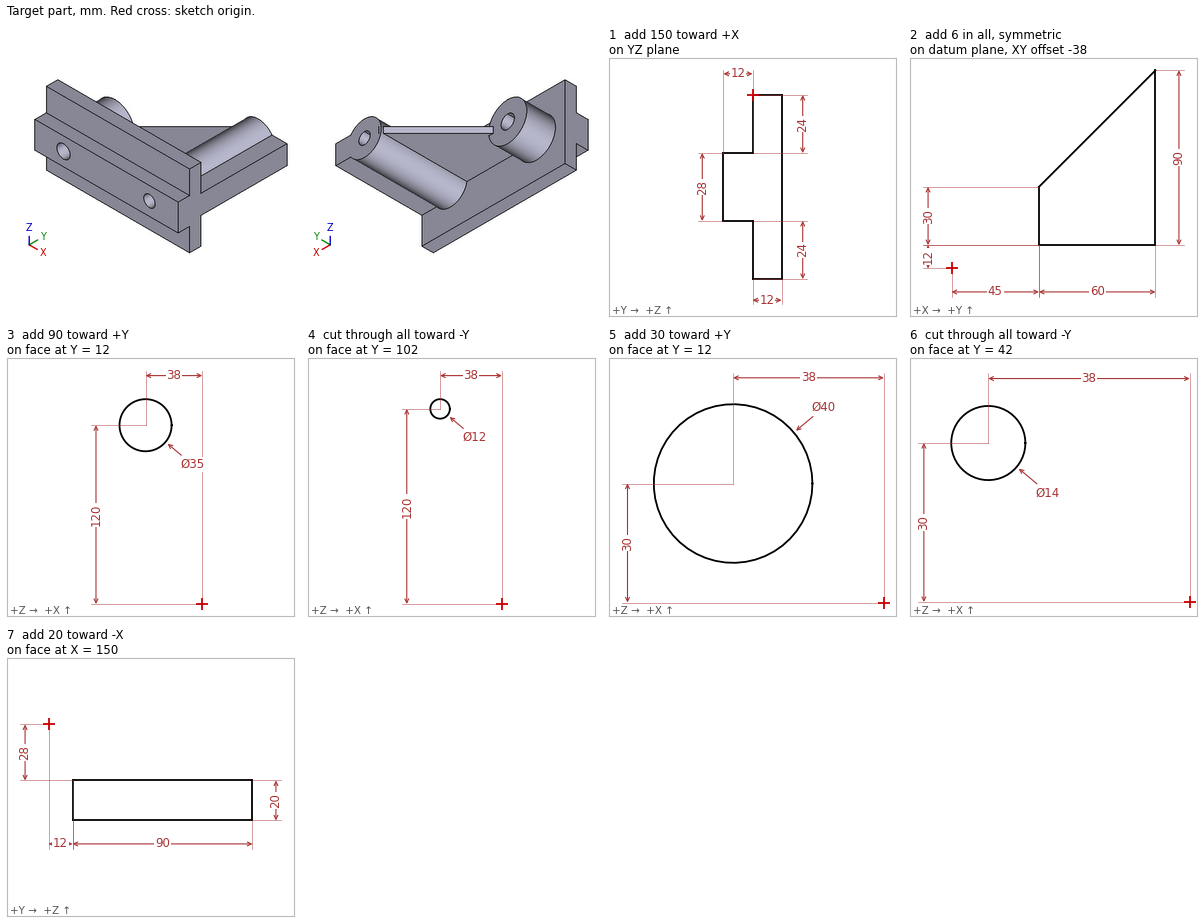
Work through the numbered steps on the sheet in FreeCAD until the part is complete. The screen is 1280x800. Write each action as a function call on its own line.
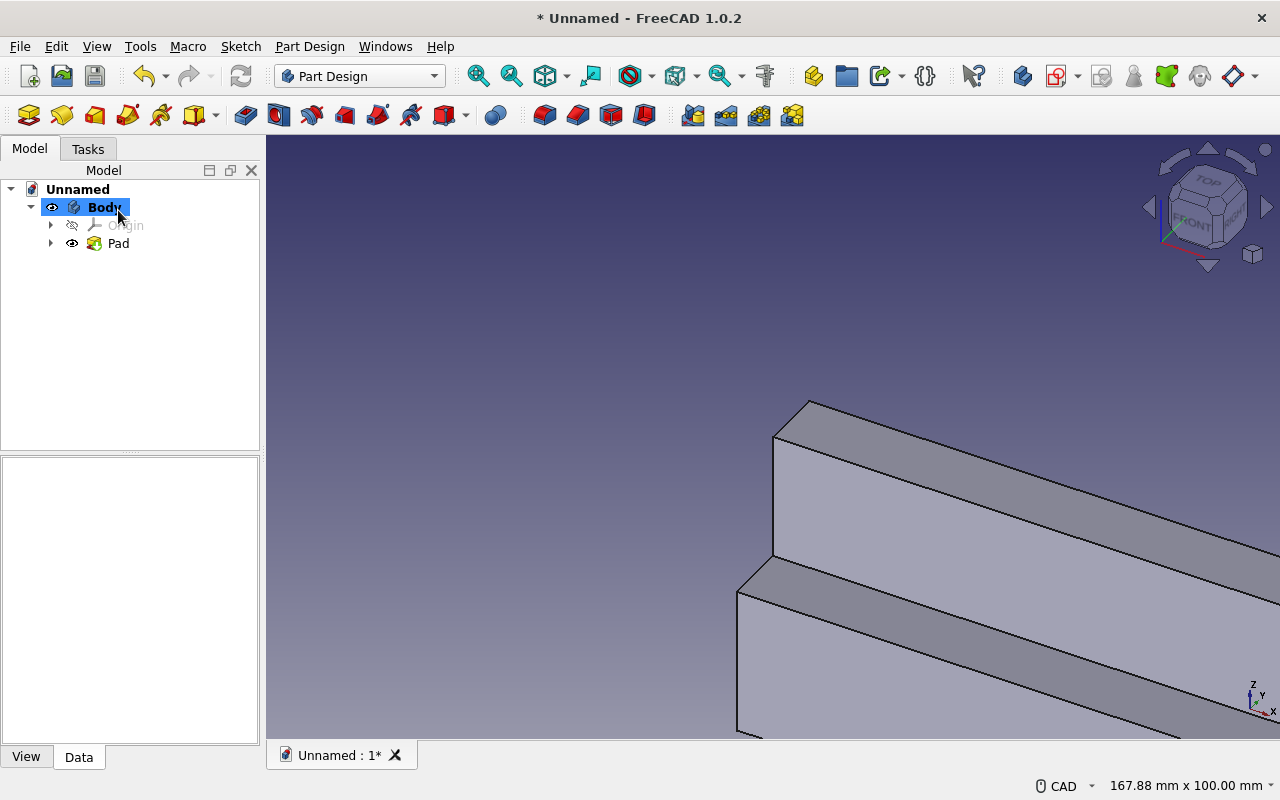
click(479, 76)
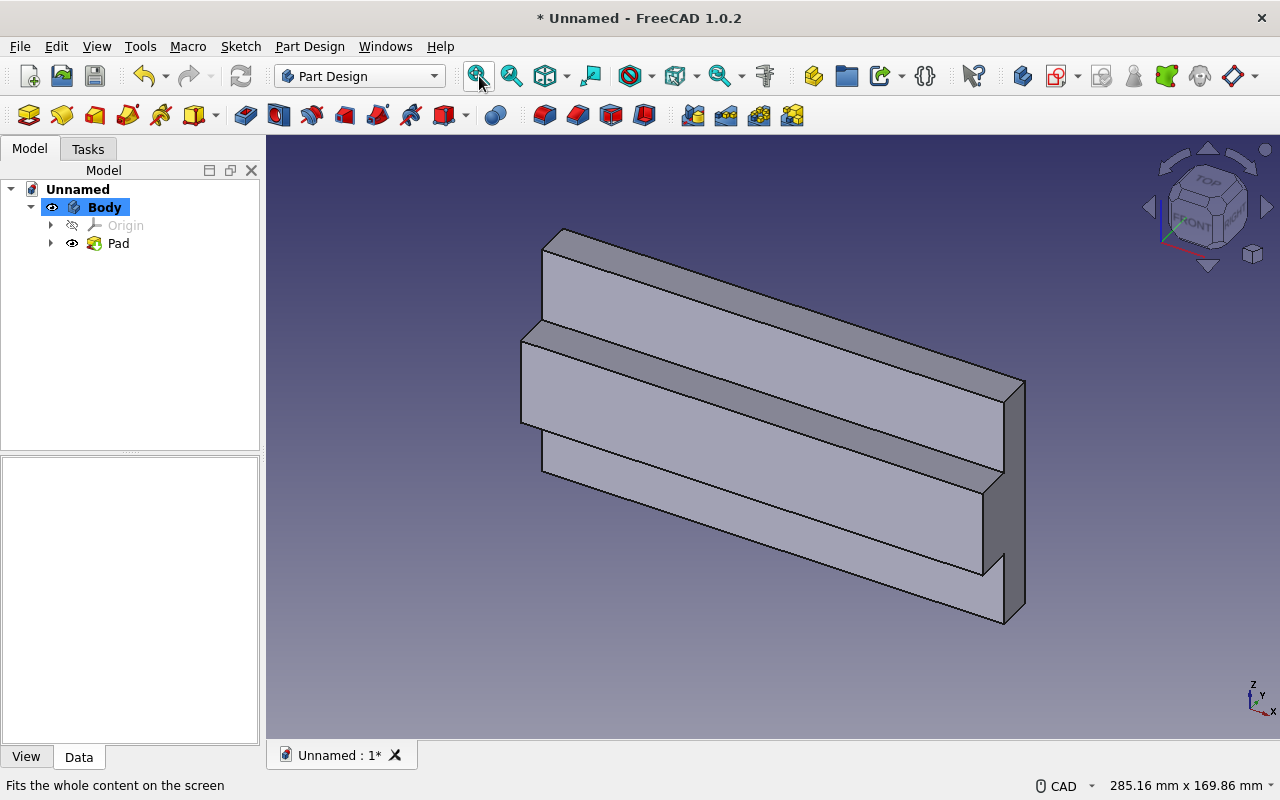
click(51, 225)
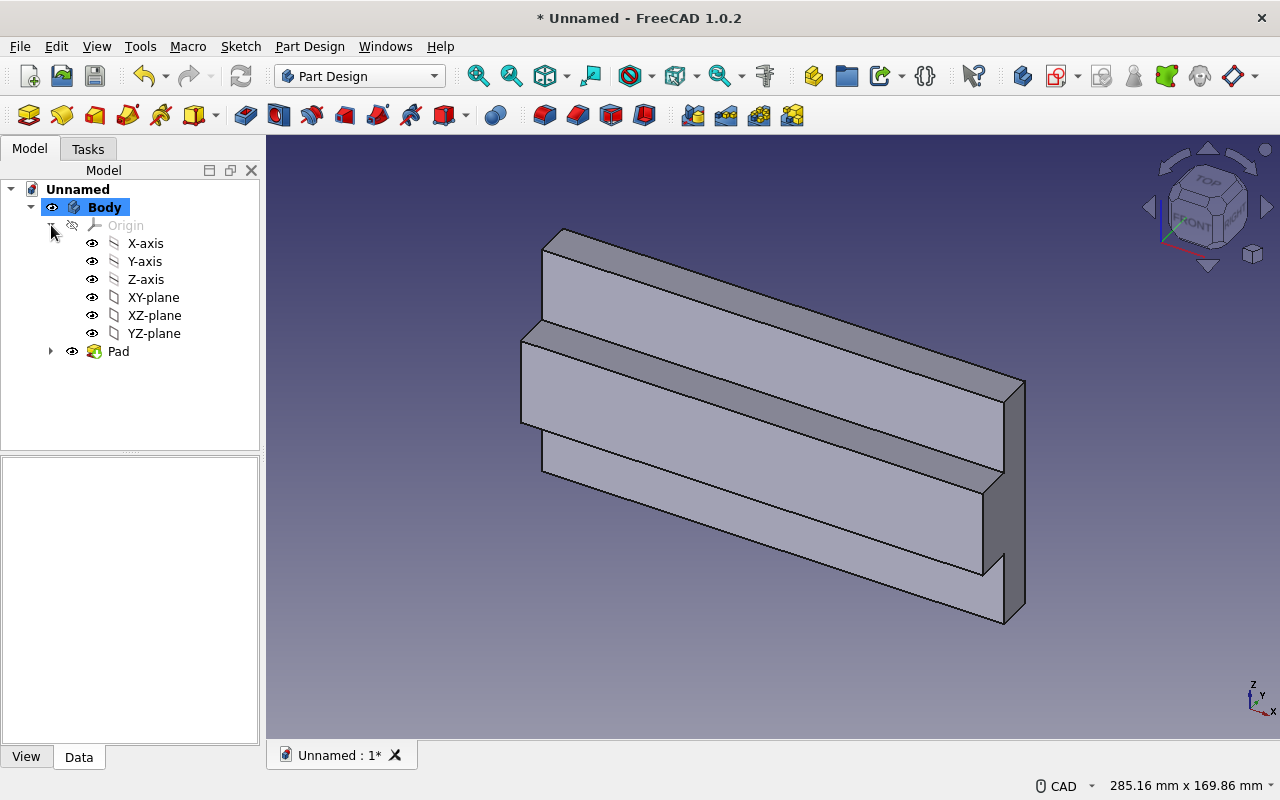
click(137, 297)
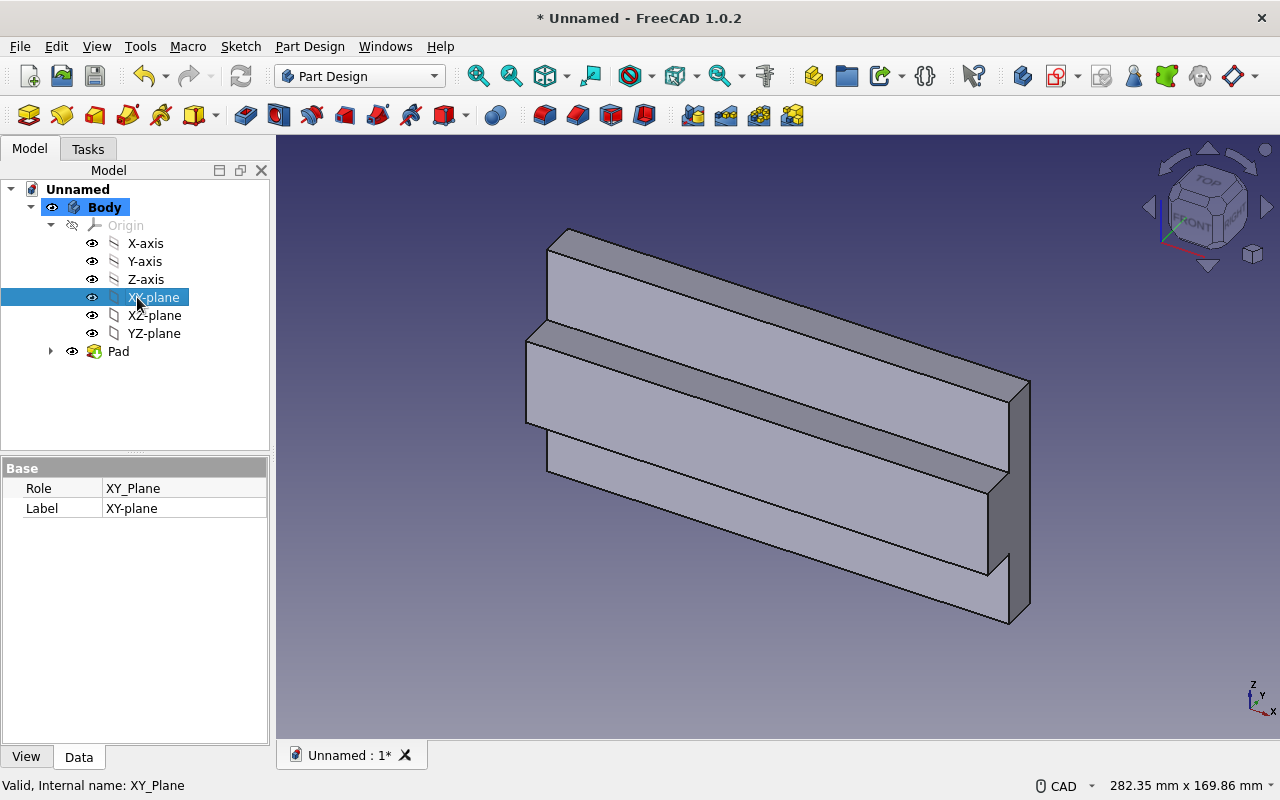
click(1232, 76)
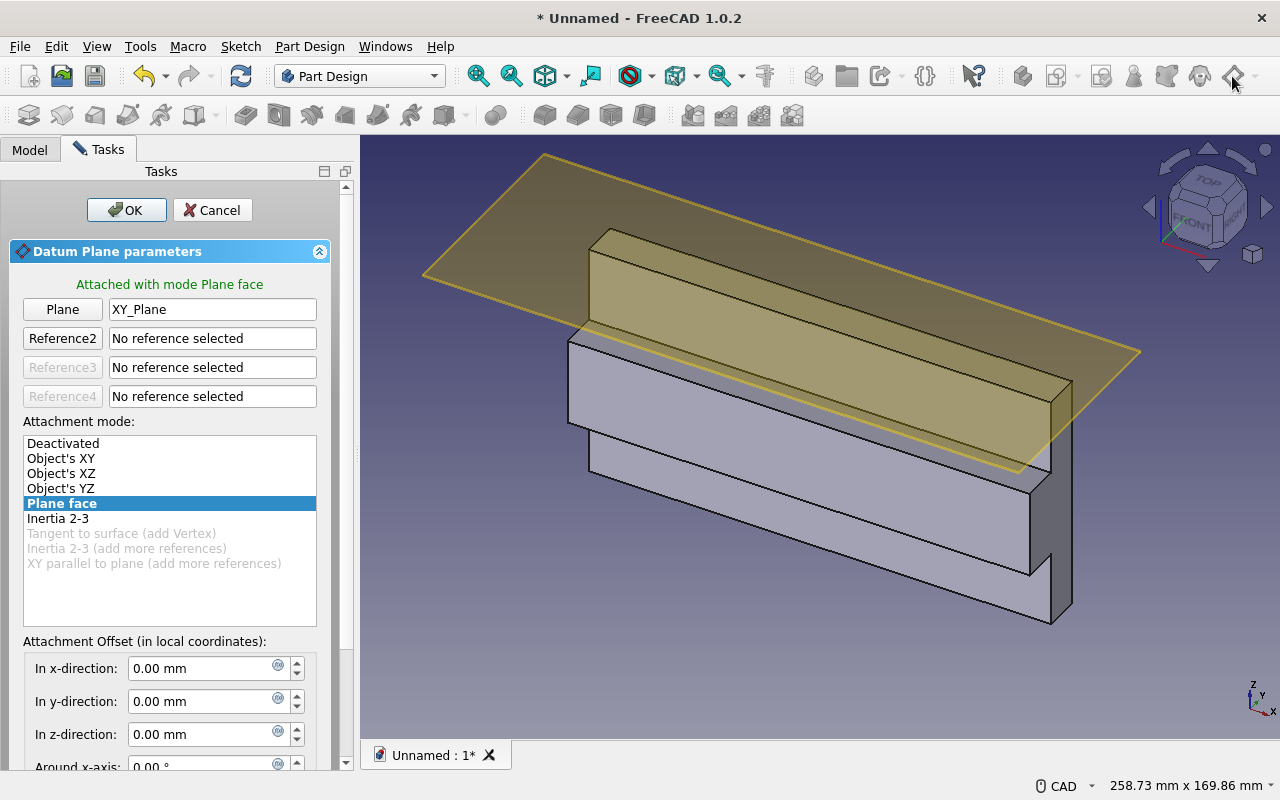
triple_click(210, 734)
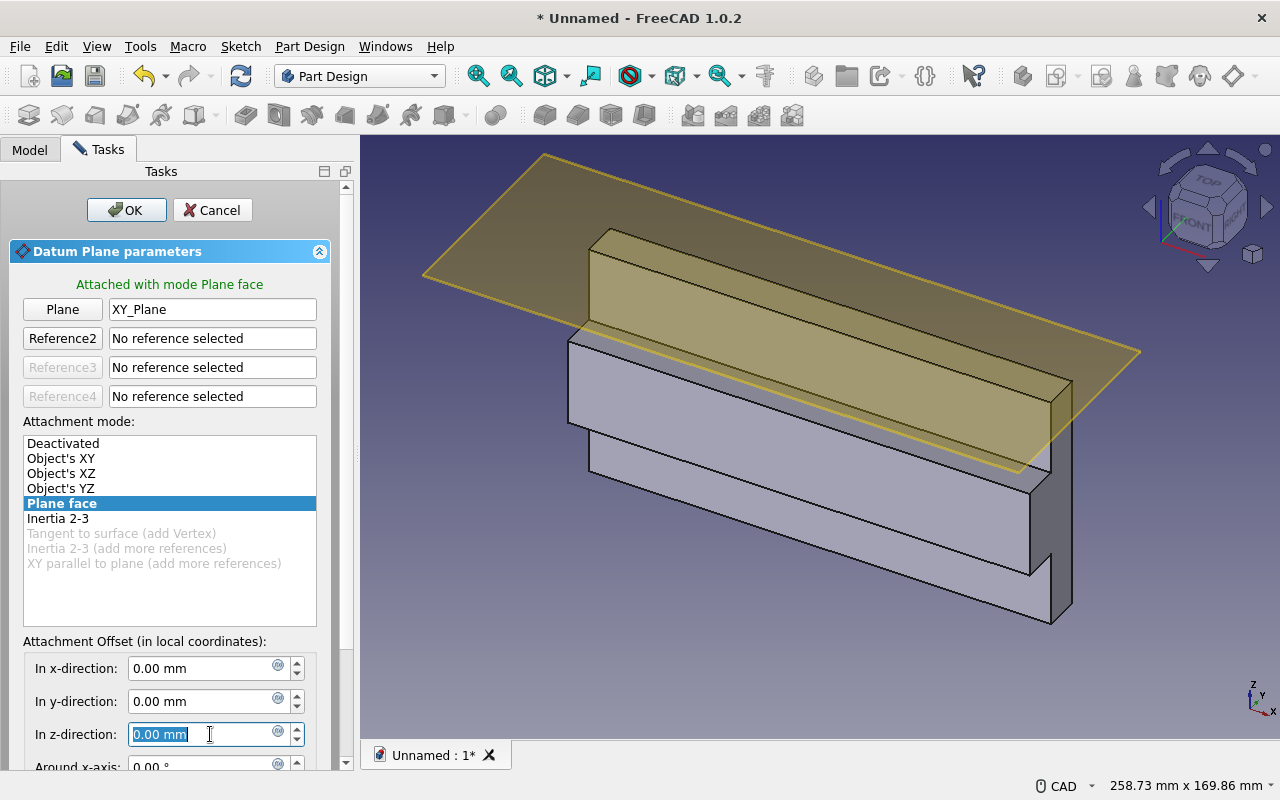
text(-38)
key(Tab)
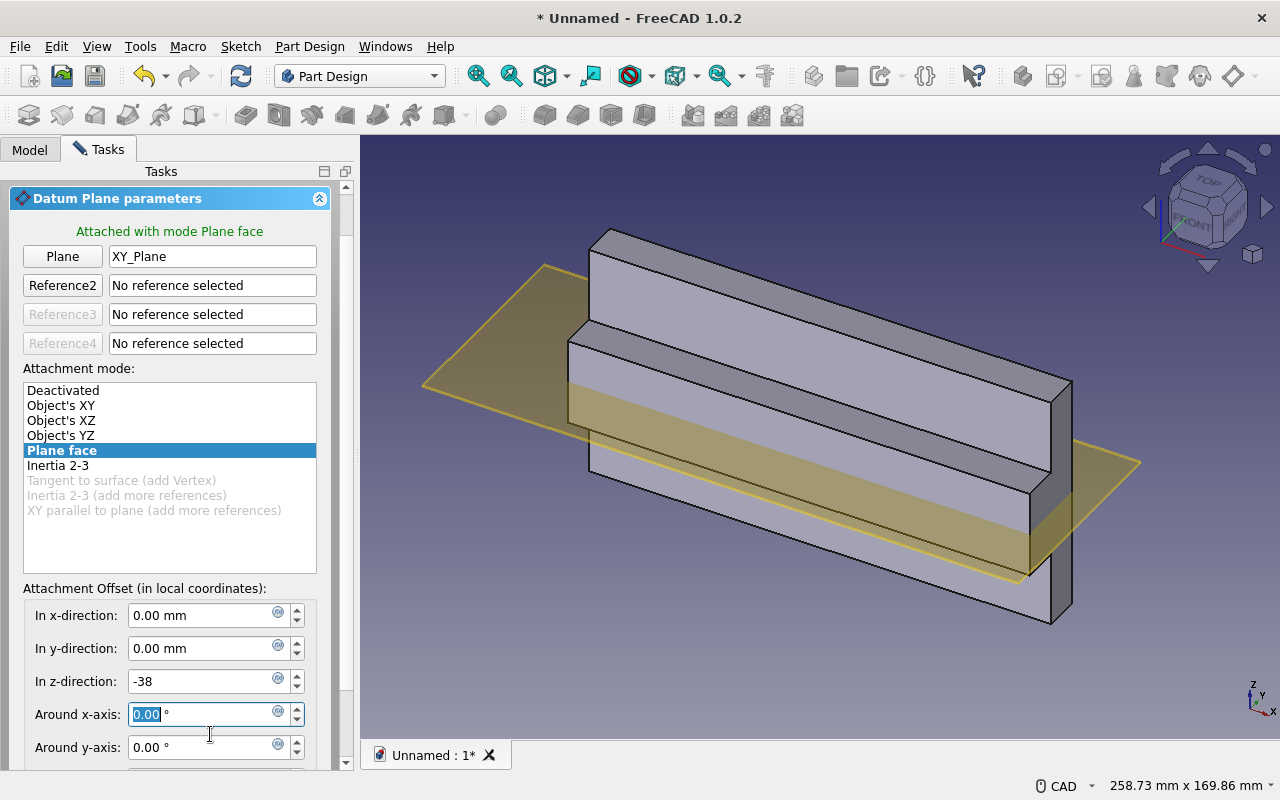
scroll(346, 476, up, 2)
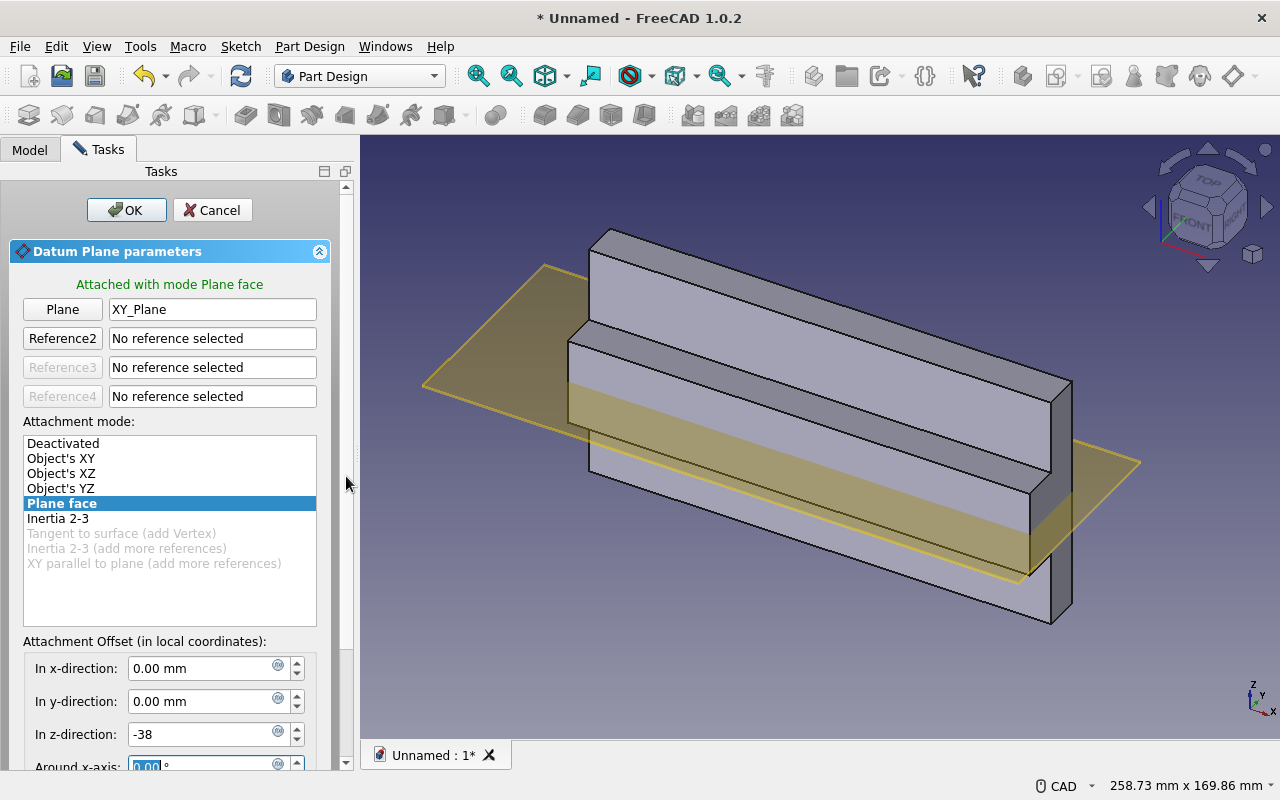
click(127, 210)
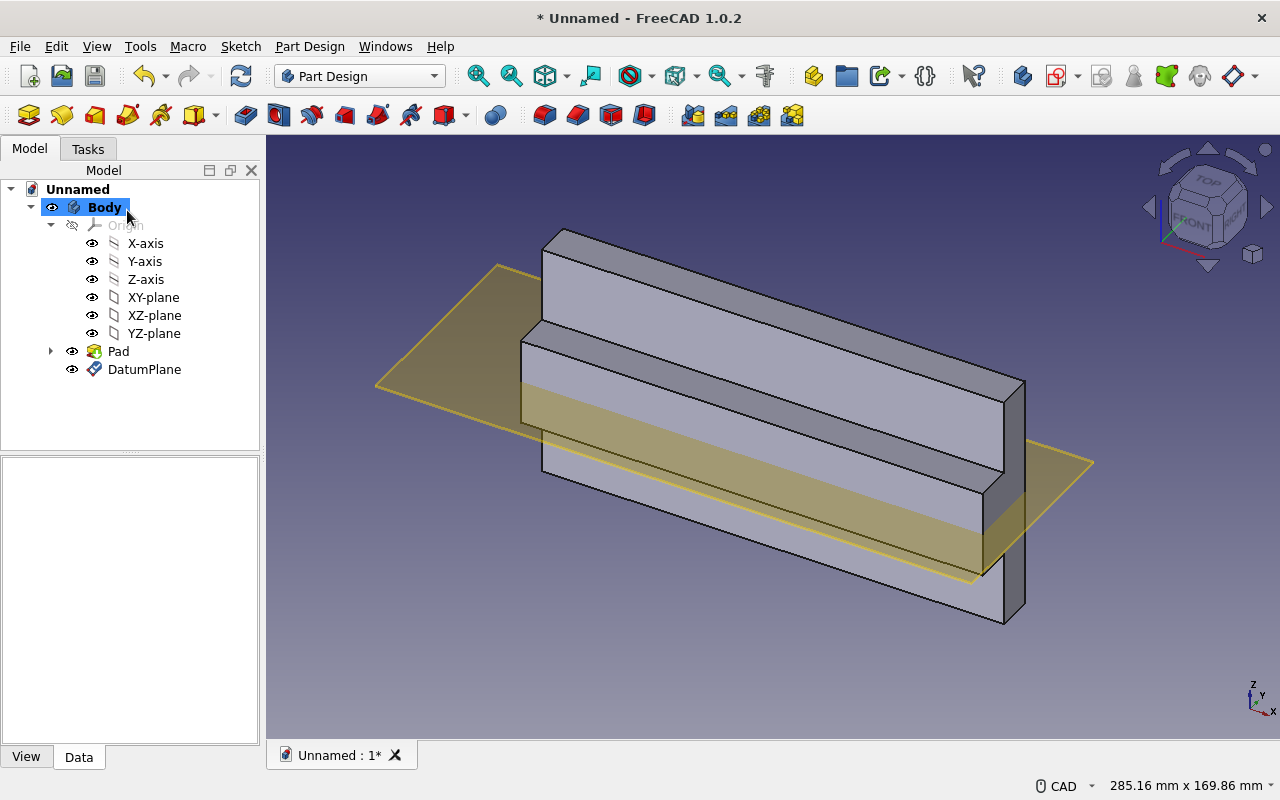
click(117, 369)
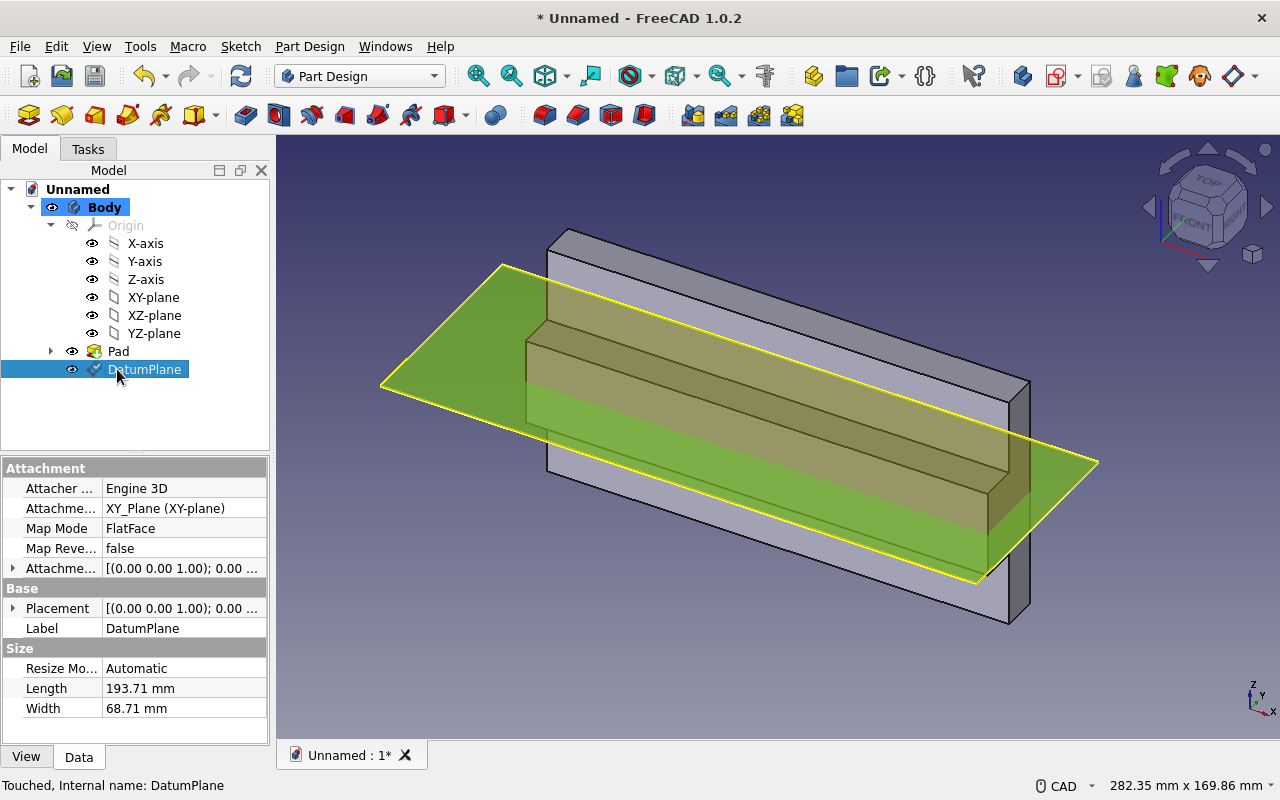
click(1056, 76)